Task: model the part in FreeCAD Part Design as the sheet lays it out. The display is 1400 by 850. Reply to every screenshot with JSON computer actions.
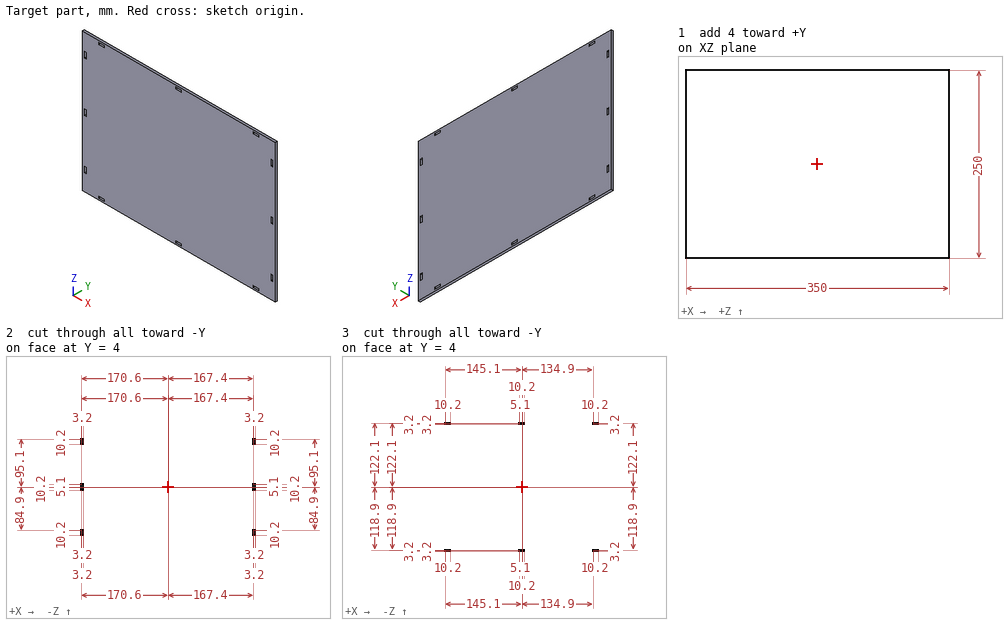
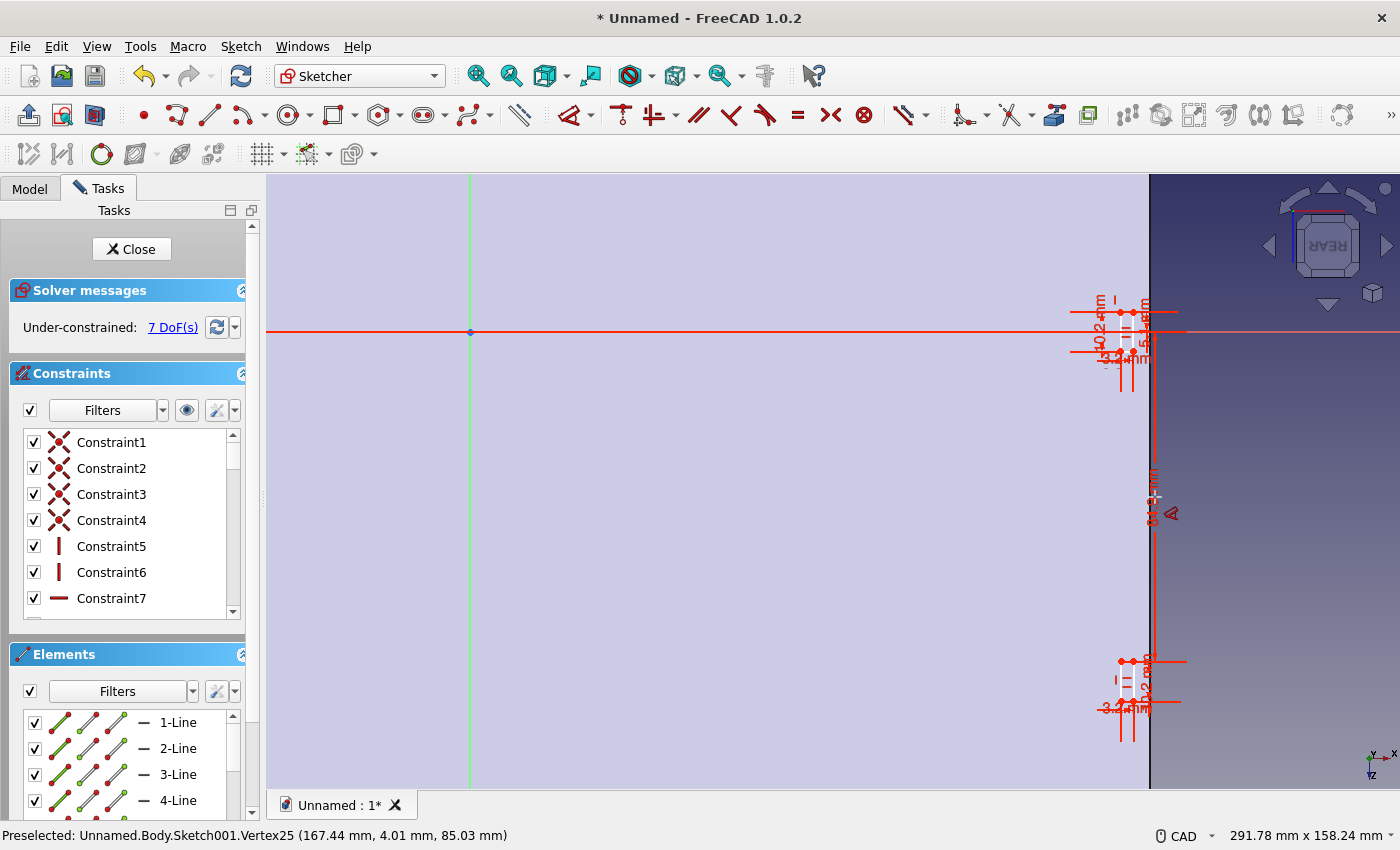
{"action": "scroll", "coordinate": [1122, 663], "scroll_direction": "down", "scroll_amount": 3}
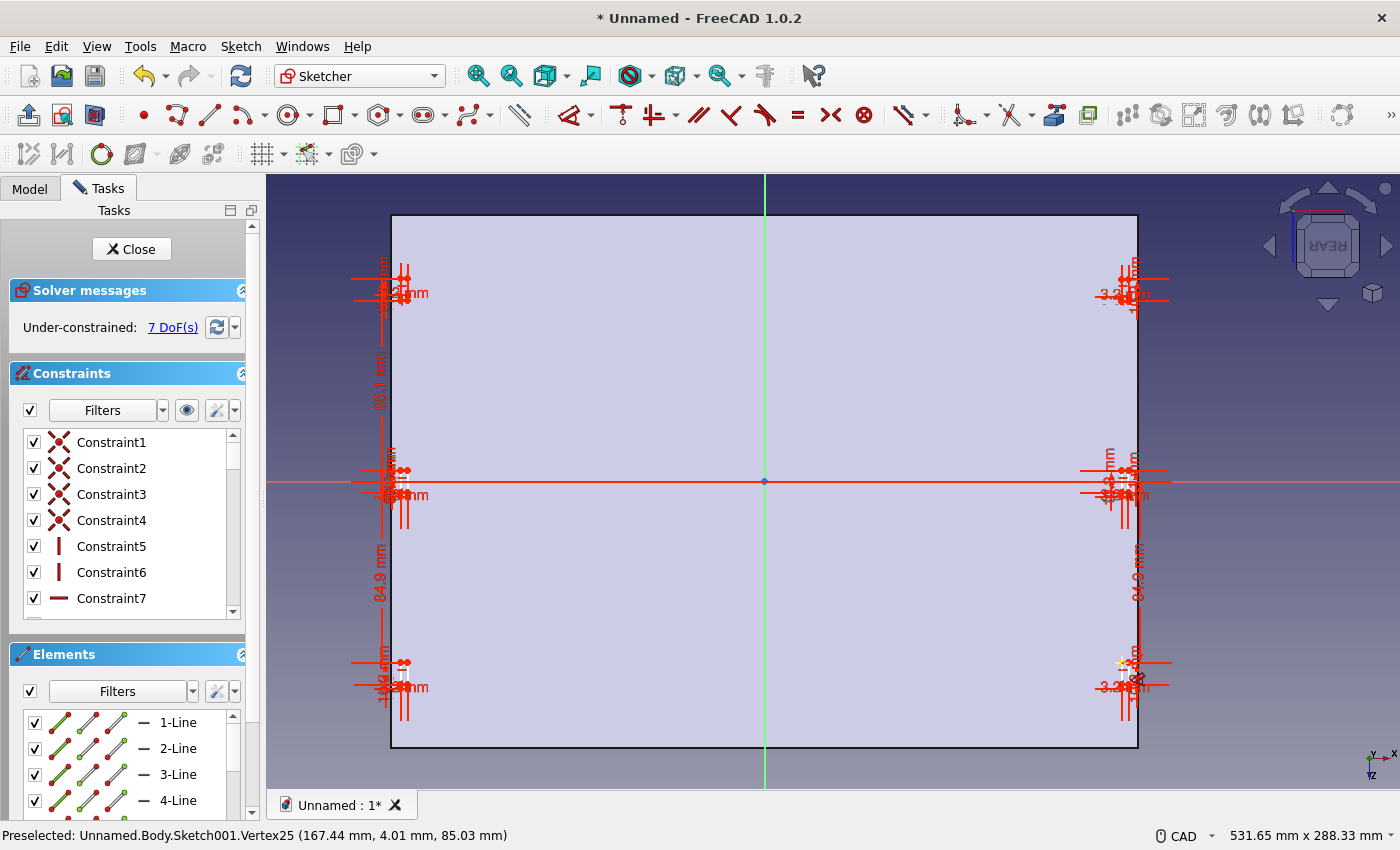
{"action": "scroll", "coordinate": [1122, 279], "scroll_direction": "up", "scroll_amount": 3}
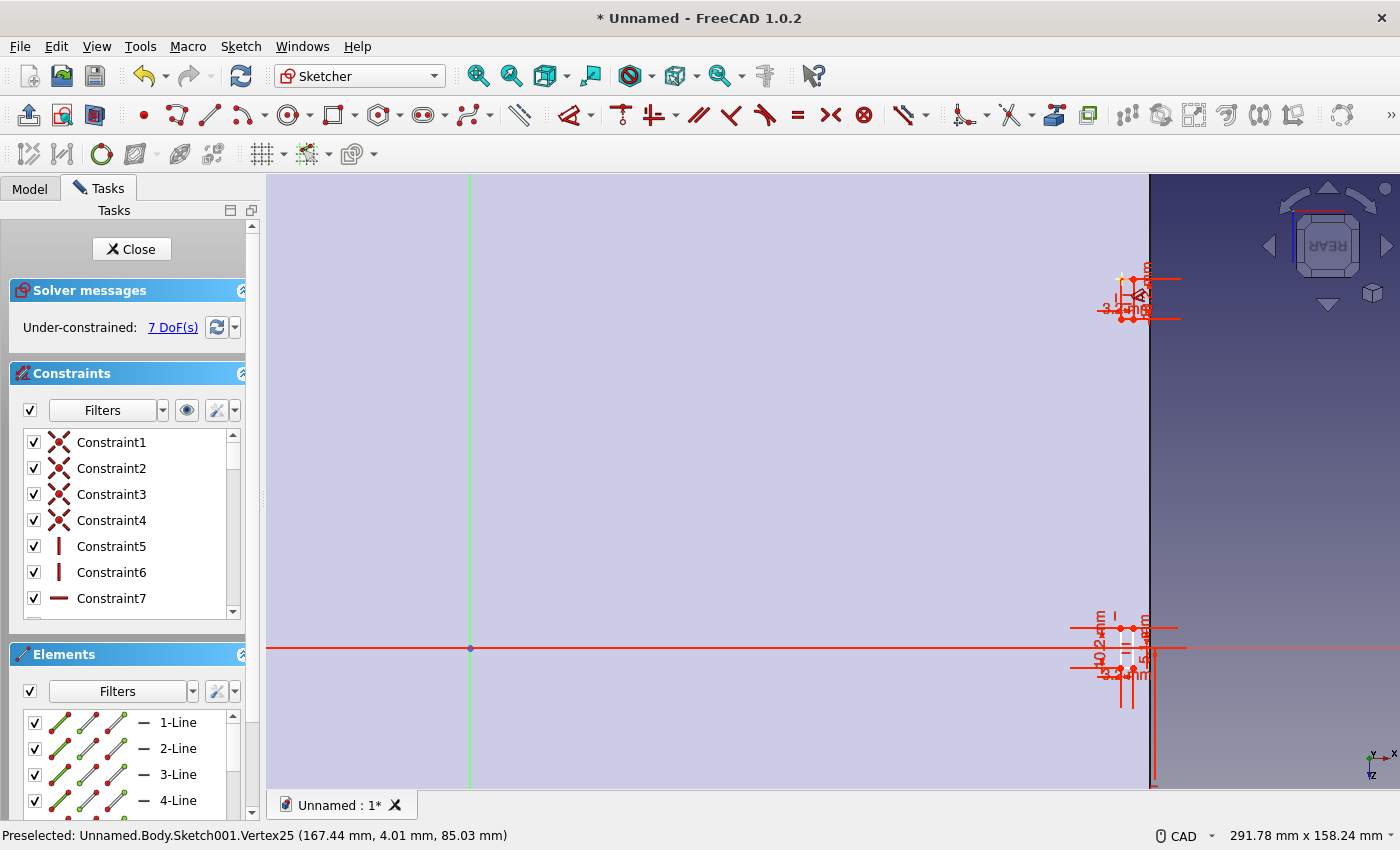
{"action": "left_click", "coordinate": [1121, 279]}
{"action": "left_click", "coordinate": [1155, 464]}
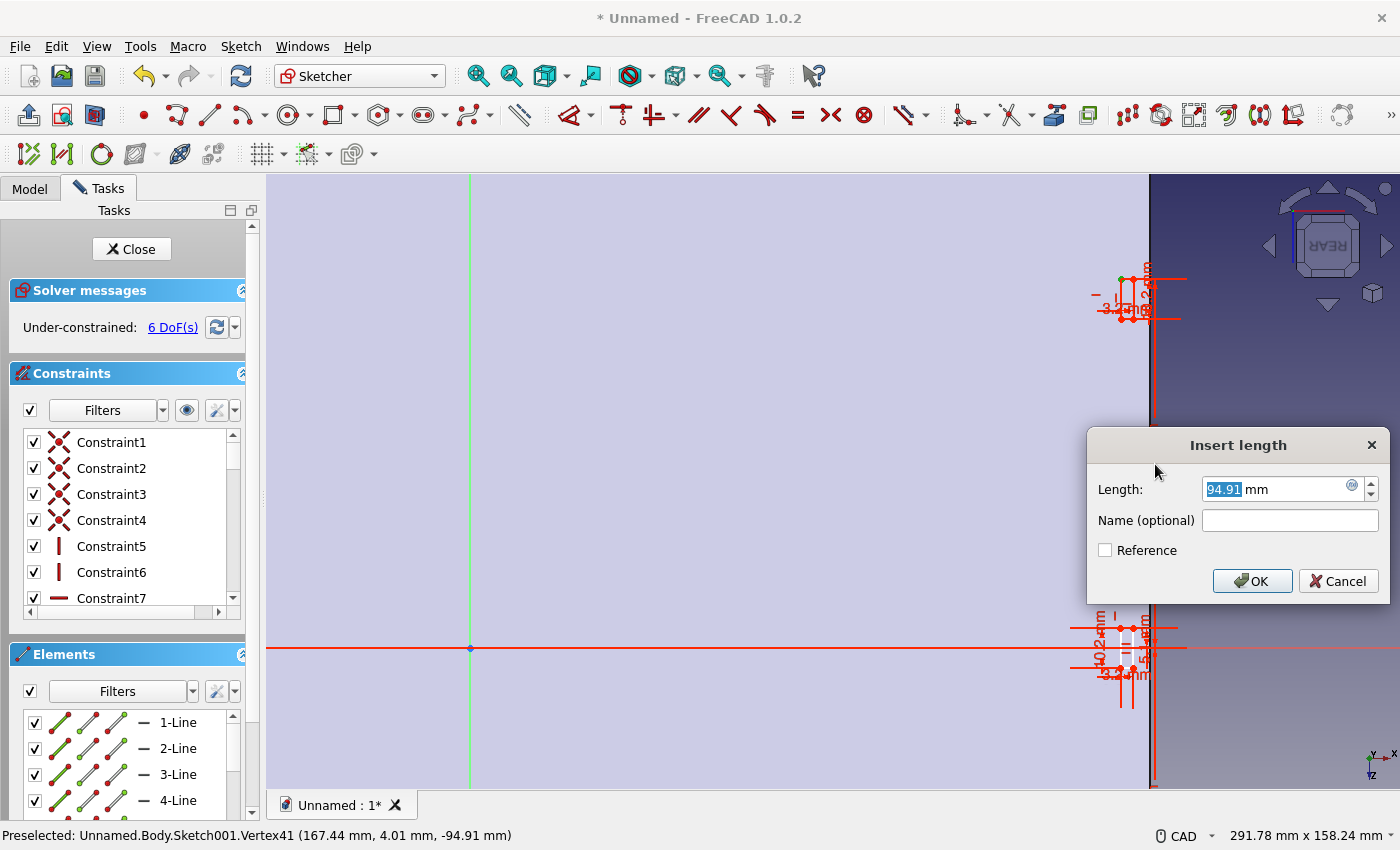
{"action": "type", "text": "95.1"}
{"action": "key", "text": "Return"}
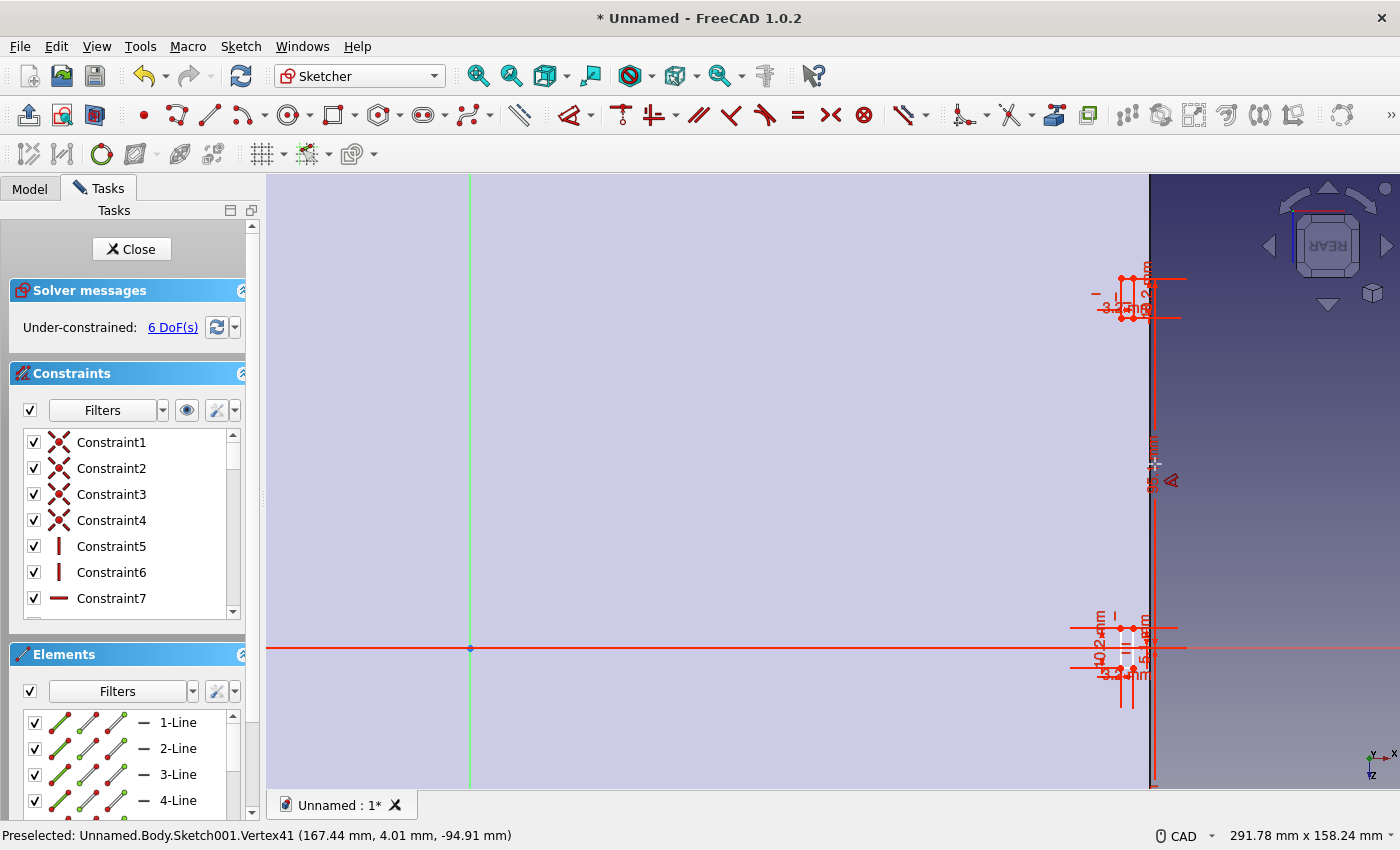
{"action": "scroll", "coordinate": [1122, 279], "scroll_direction": "down", "scroll_amount": 3}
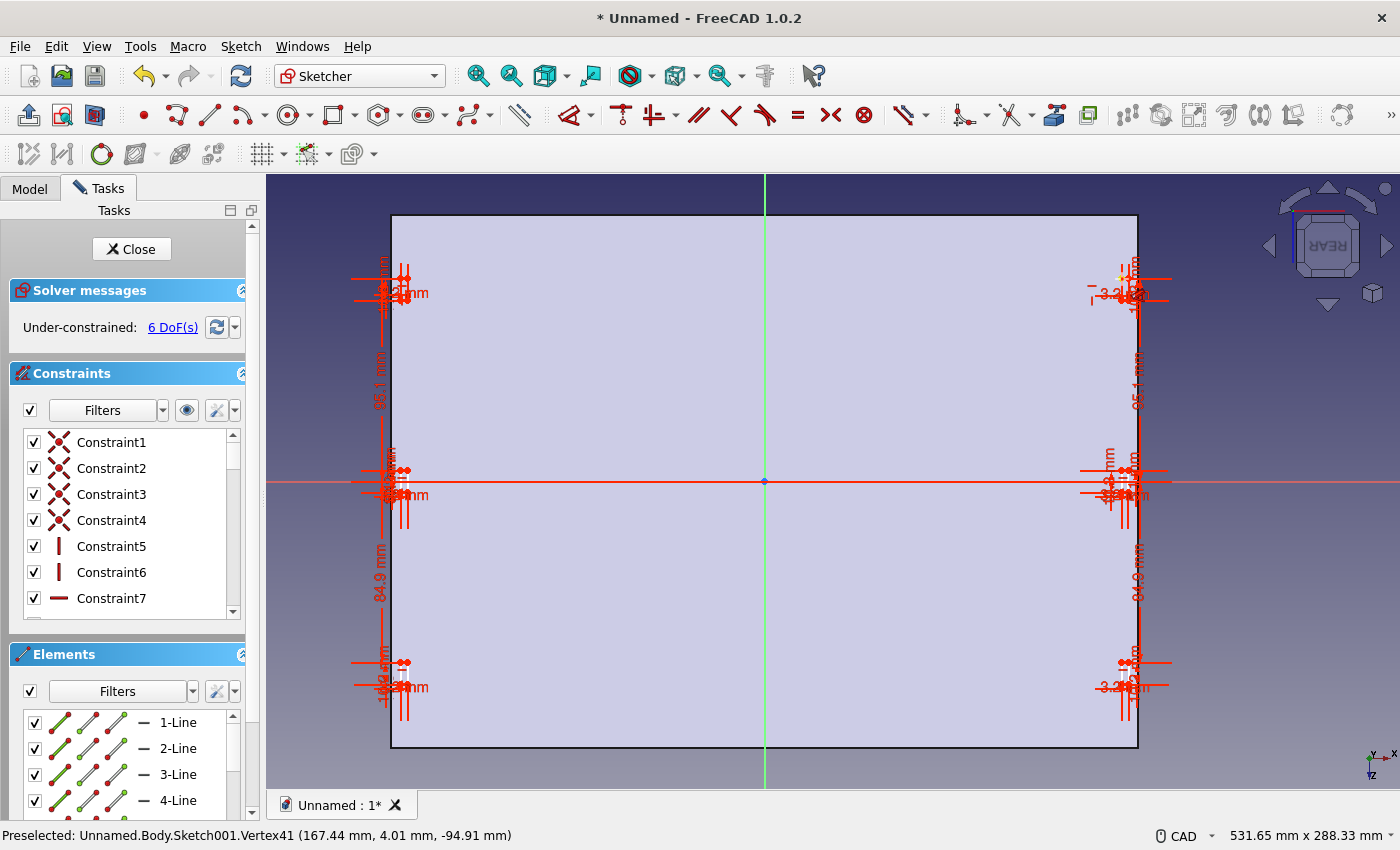
{"action": "scroll", "coordinate": [401, 279], "scroll_direction": "up", "scroll_amount": 3}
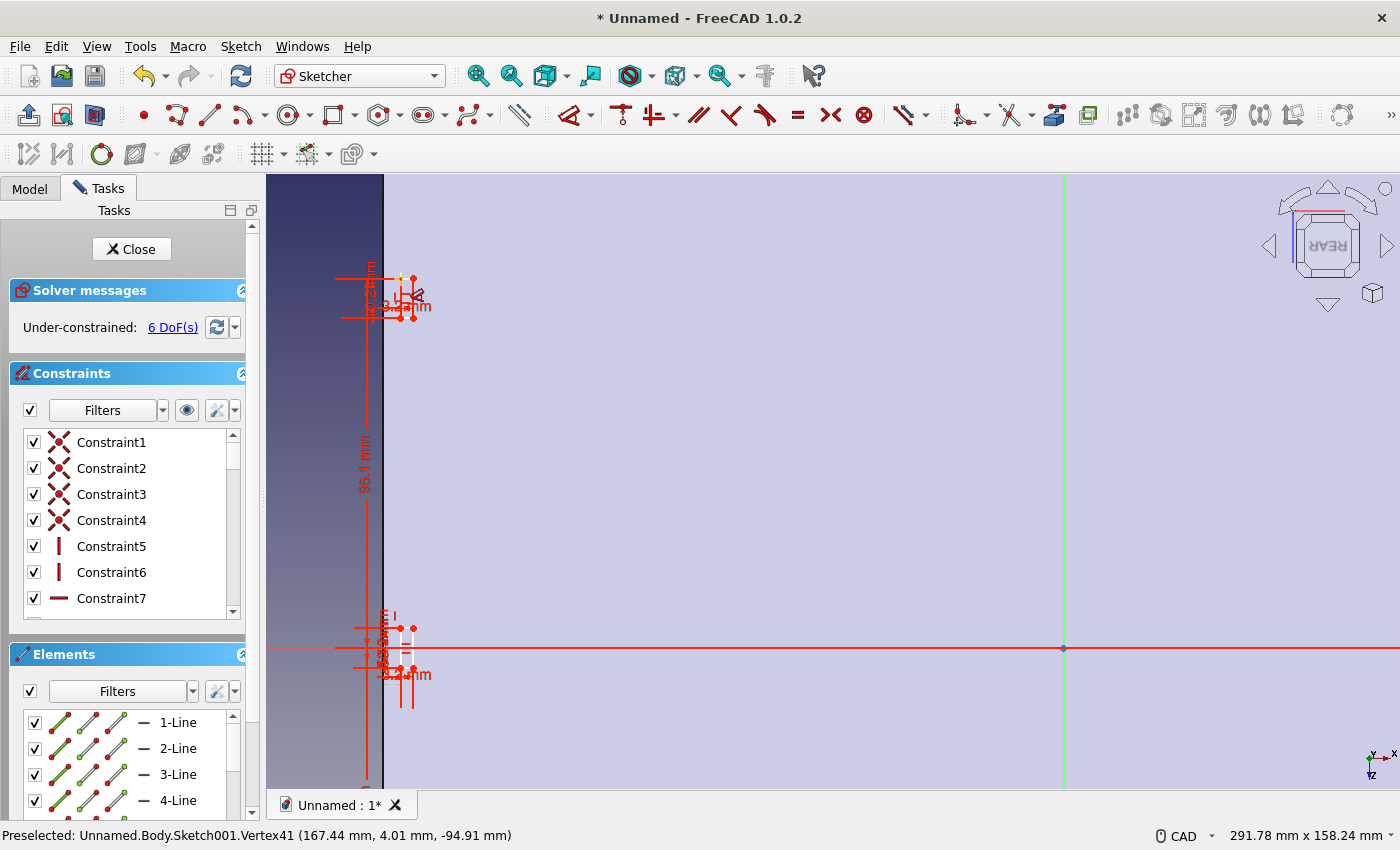
{"action": "left_click", "coordinate": [401, 279]}
{"action": "left_click", "coordinate": [732, 245]}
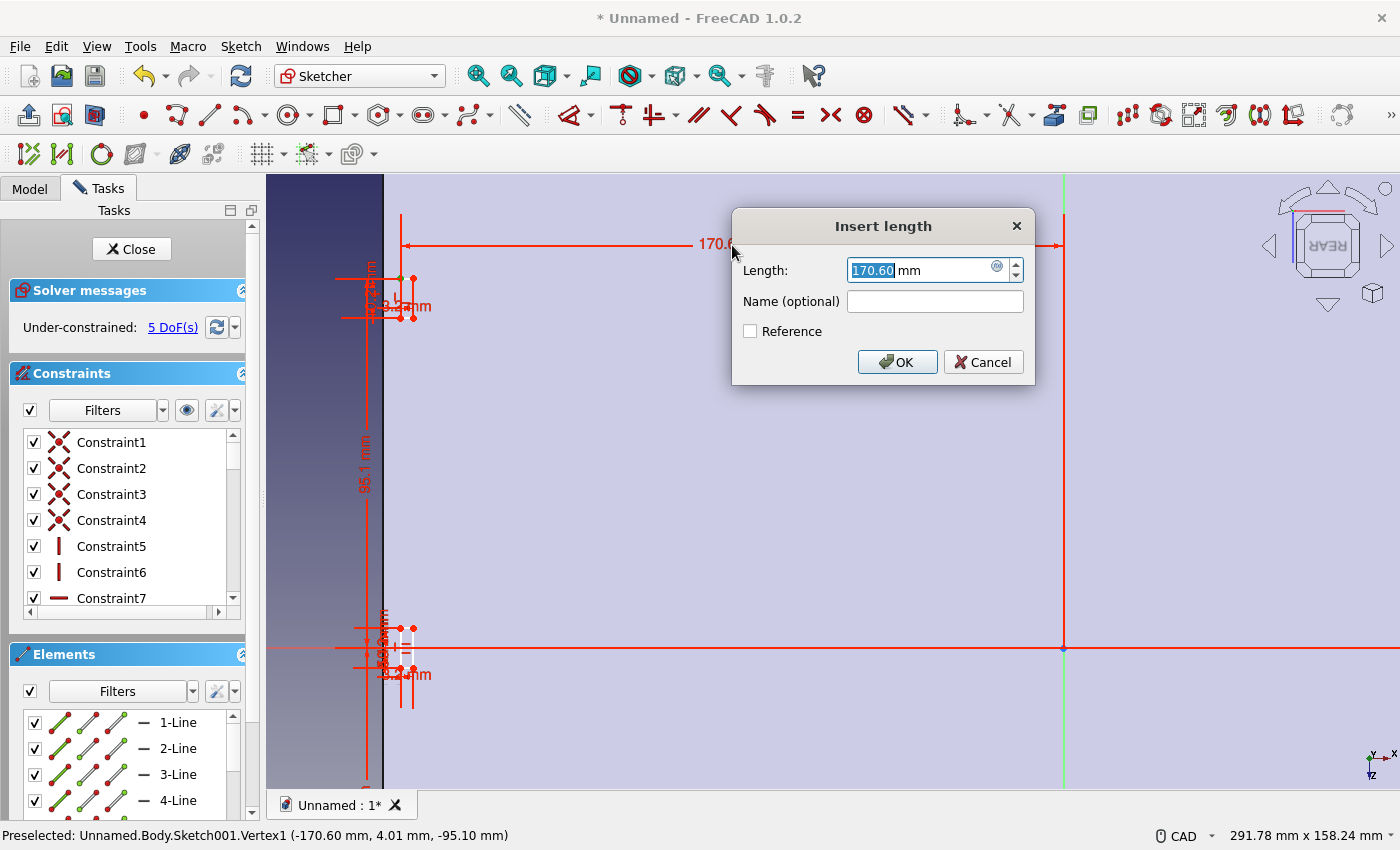
{"action": "type", "text": "170.6"}
{"action": "key", "text": "Return"}